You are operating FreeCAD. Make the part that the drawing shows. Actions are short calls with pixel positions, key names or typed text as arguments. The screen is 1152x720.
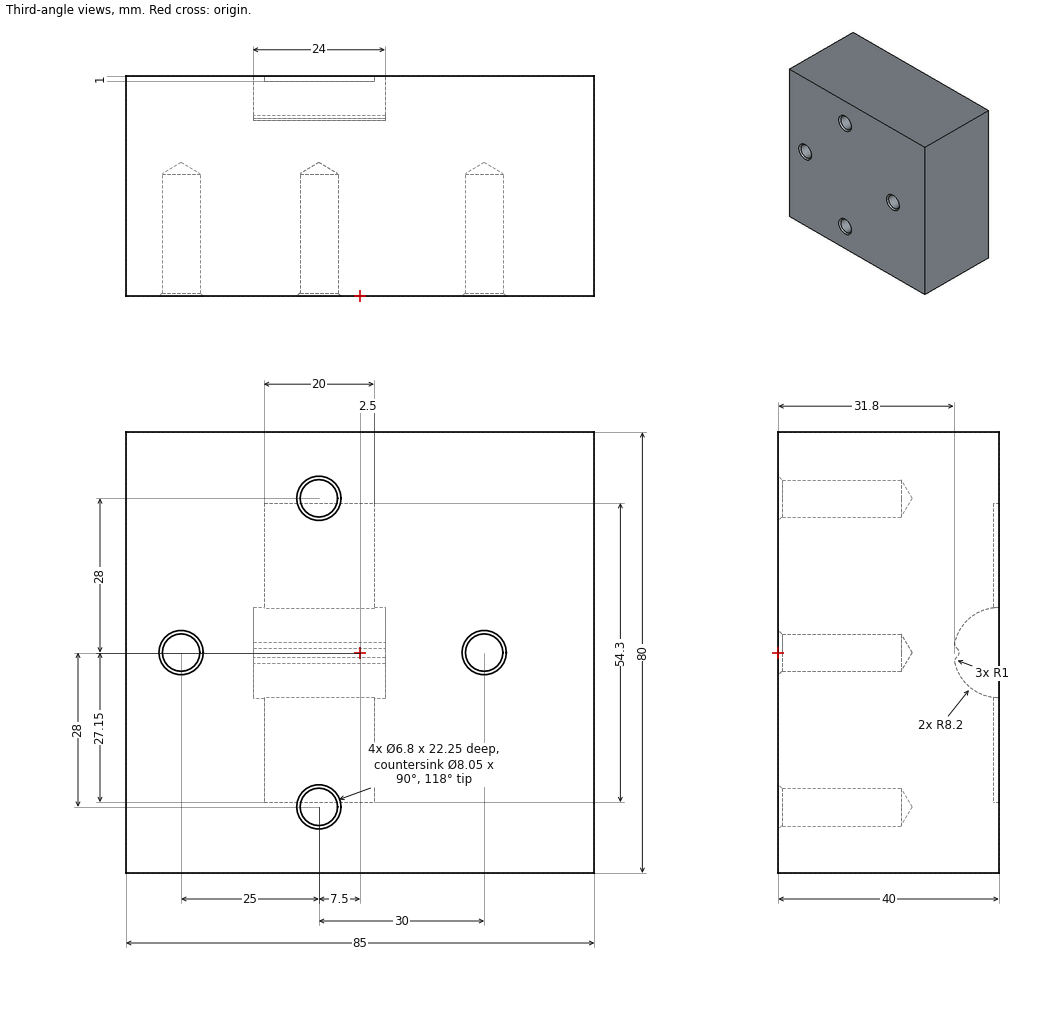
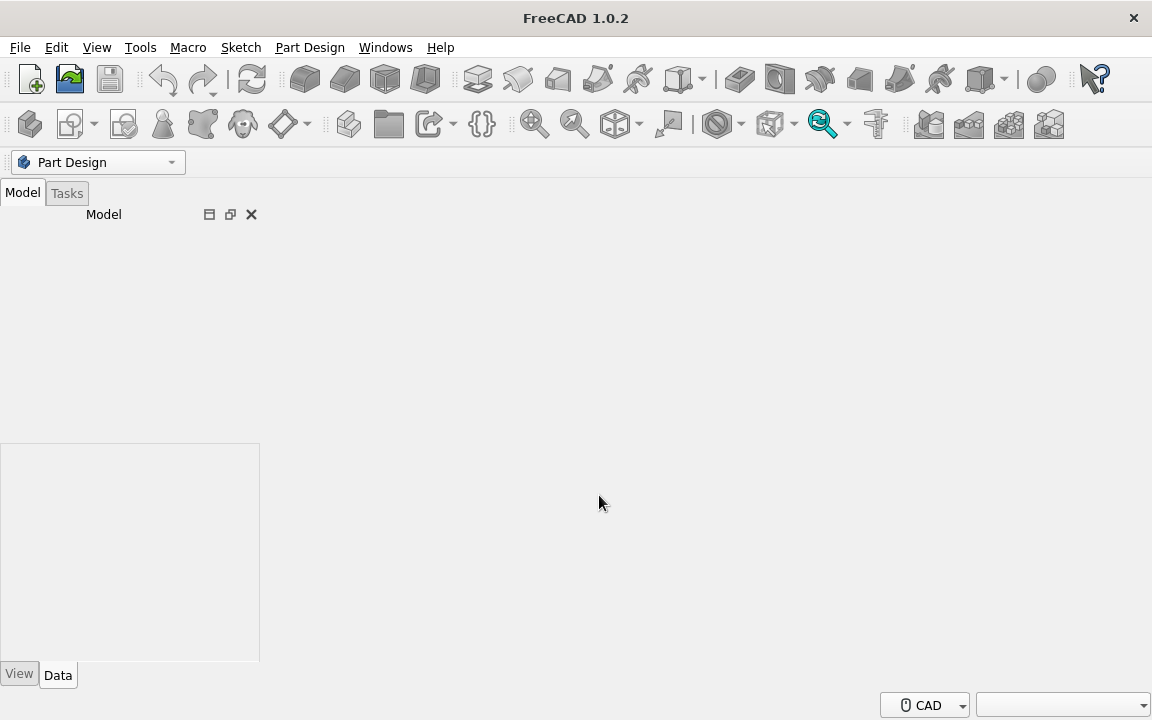
click(30, 80)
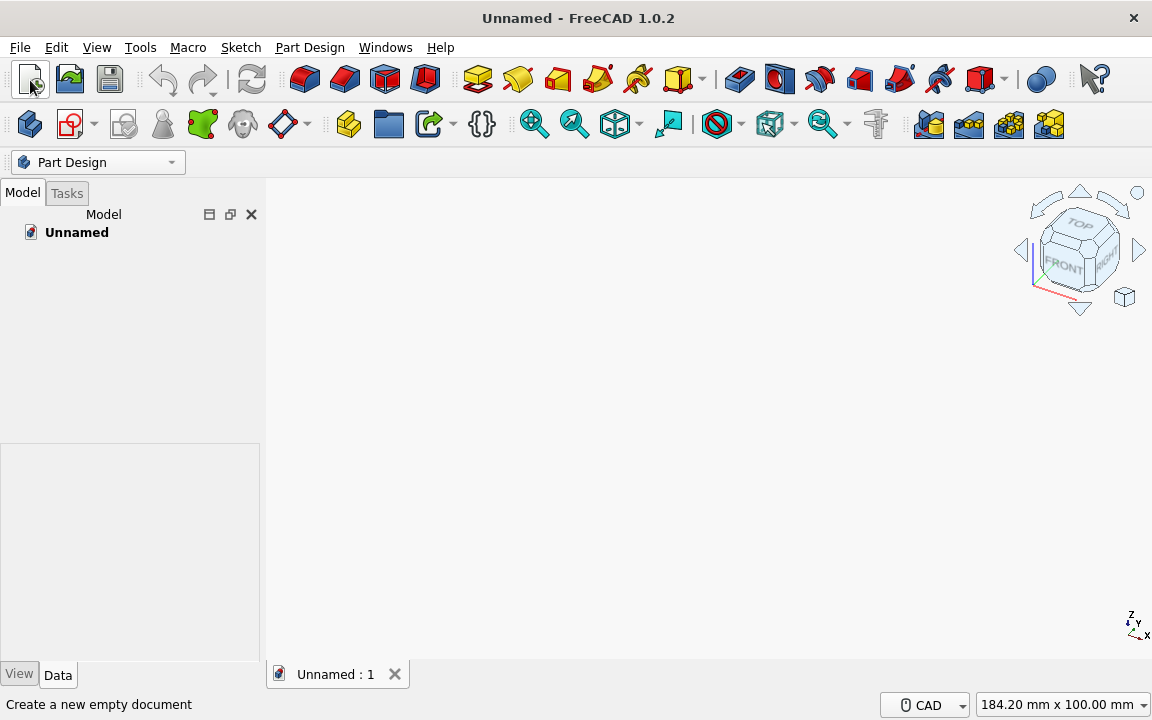
click(70, 124)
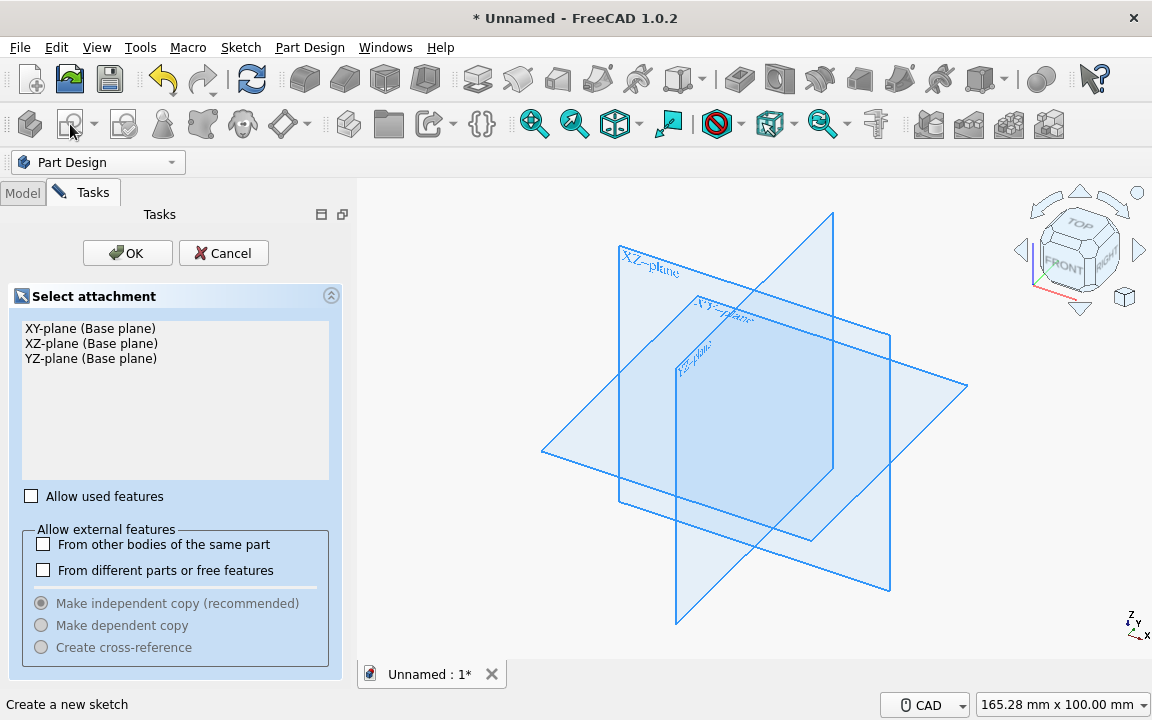
click(82, 344)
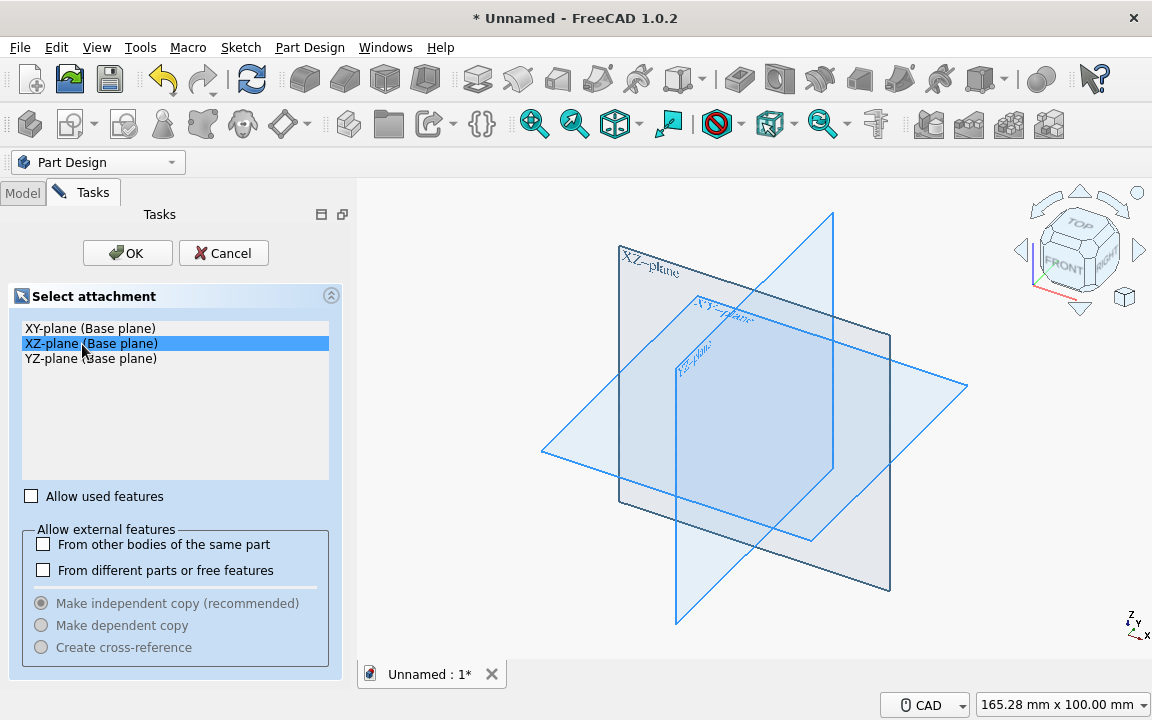
click(128, 253)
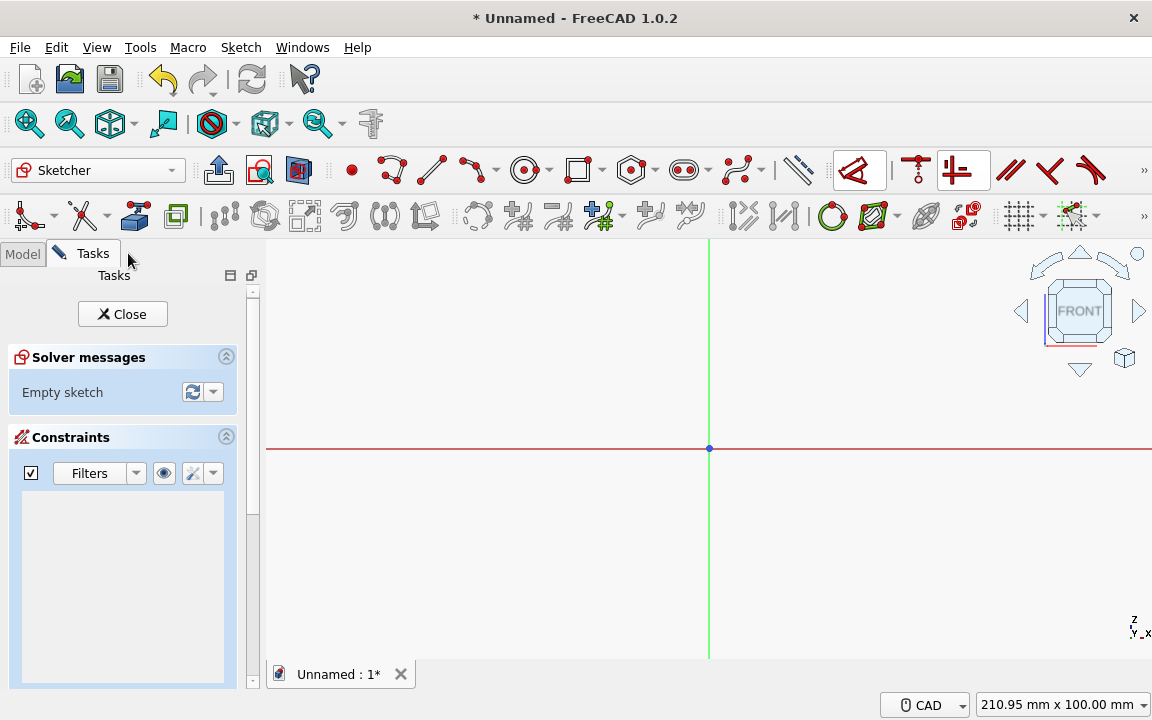
scroll(331, 449, down, 1)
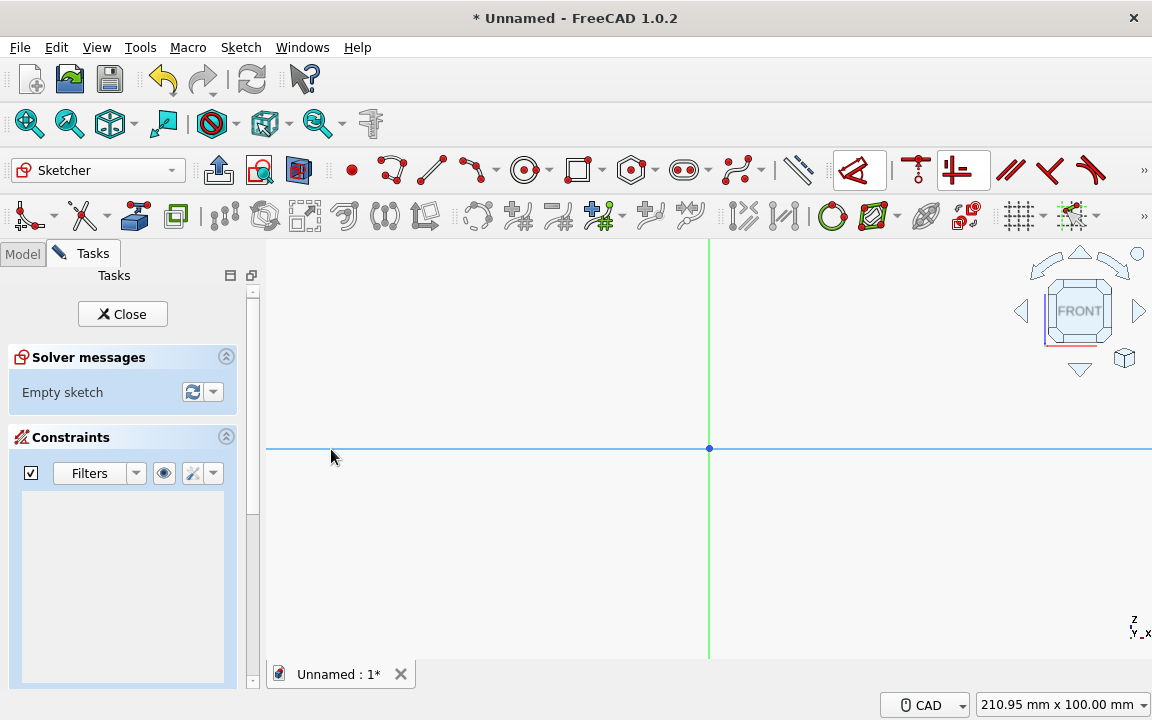
click(604, 170)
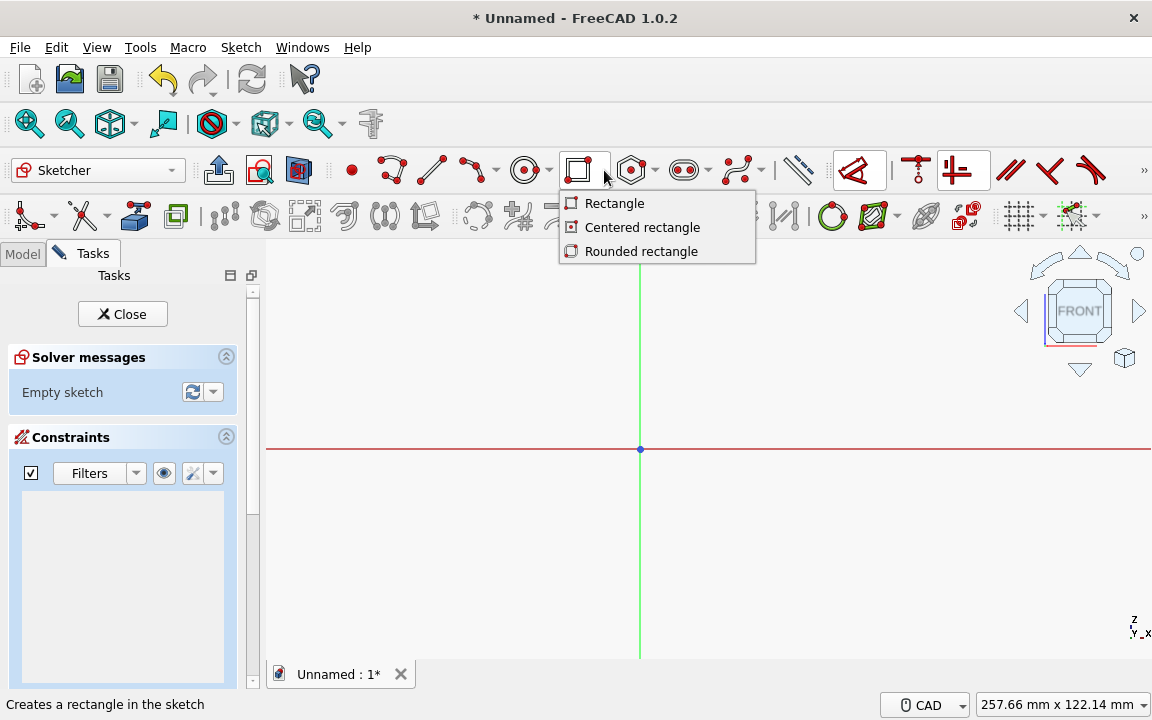
click(658, 227)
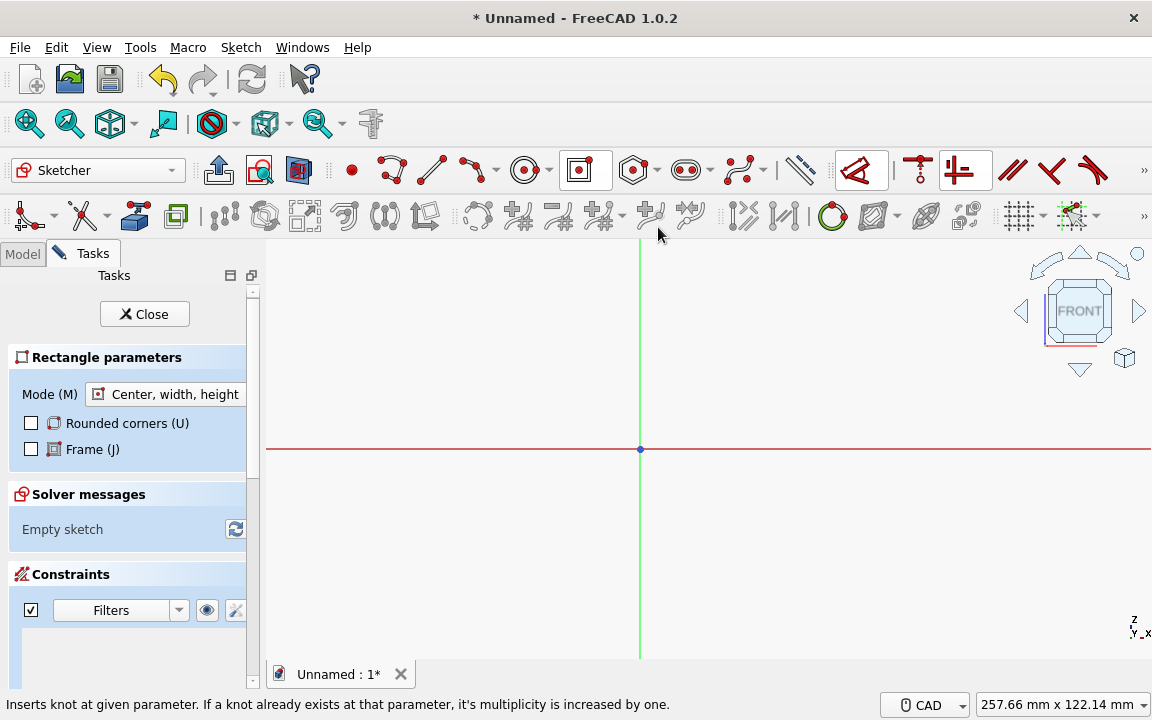
click(640, 449)
move(787, 312)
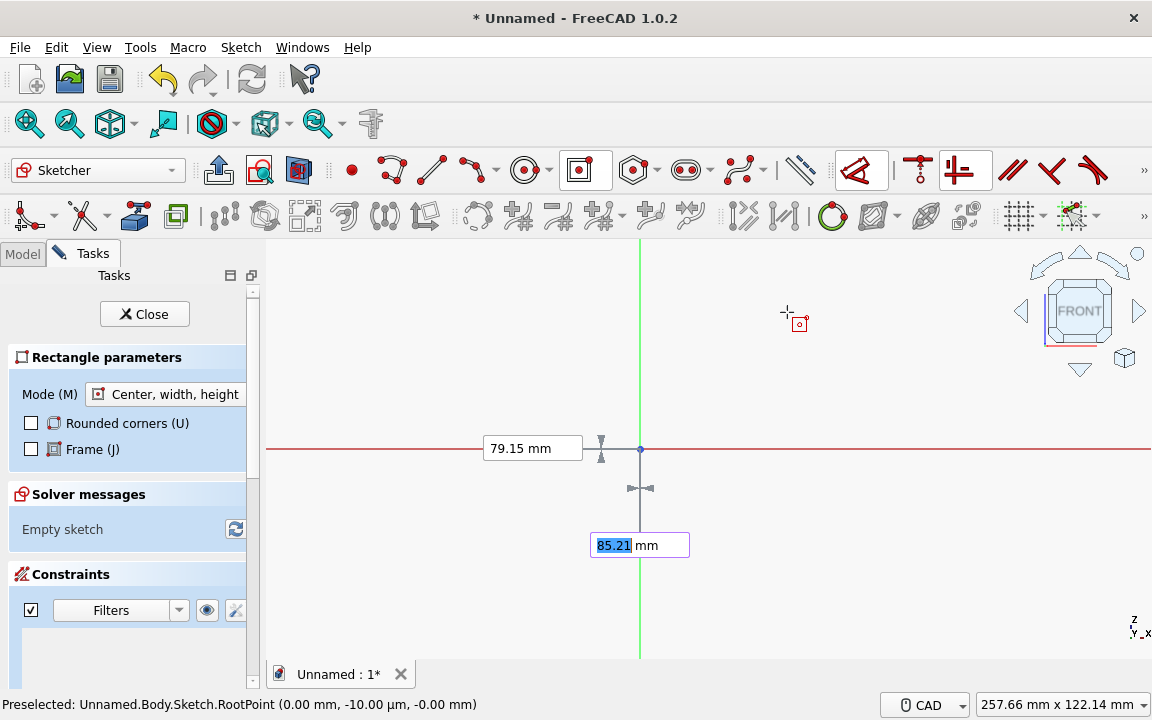
text(85)
key(Tab)
text(80)
key(Return)
key(Escape)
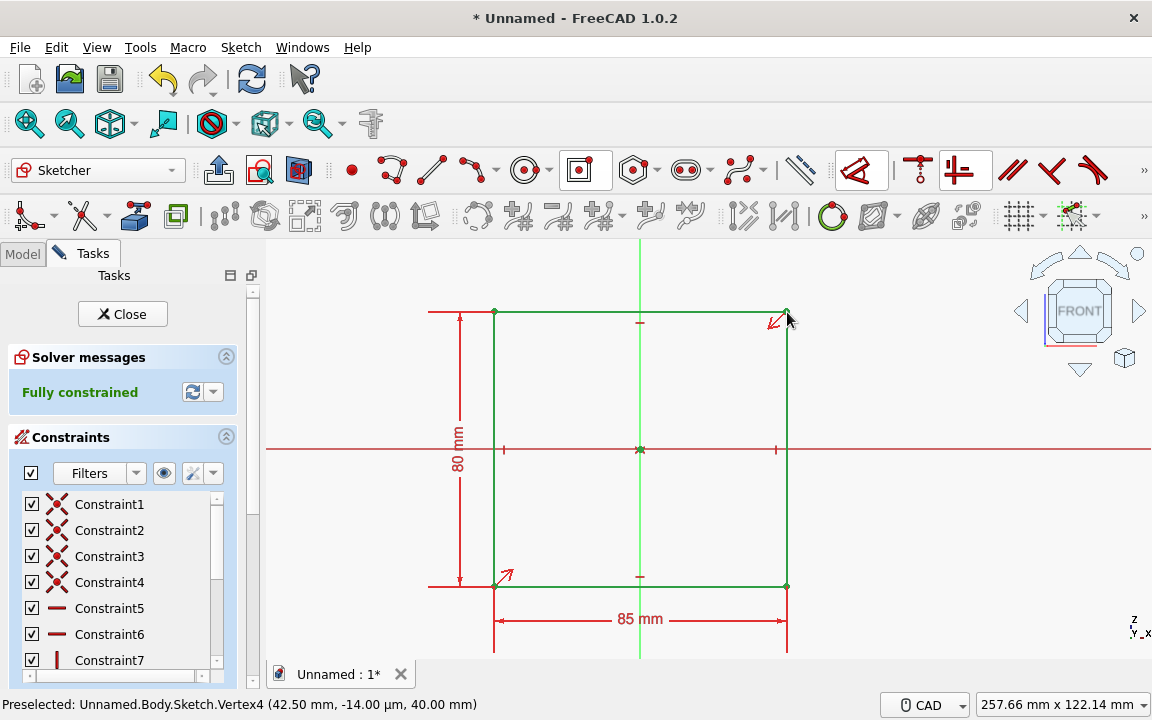
click(123, 314)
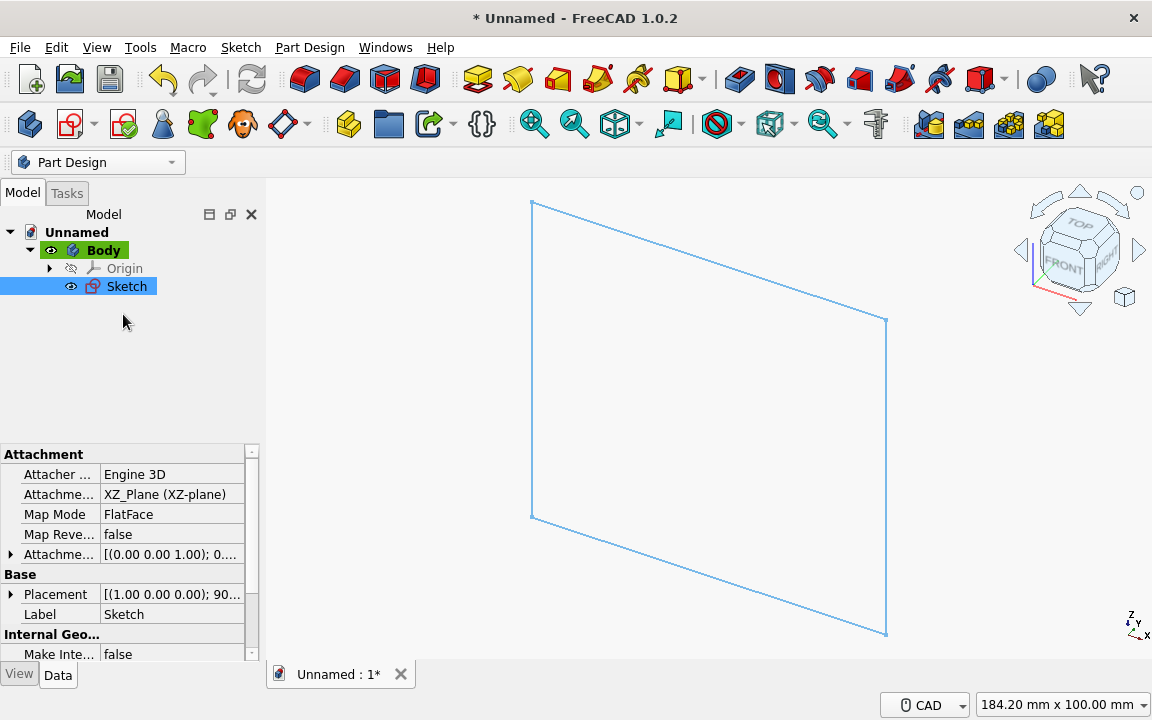
click(478, 80)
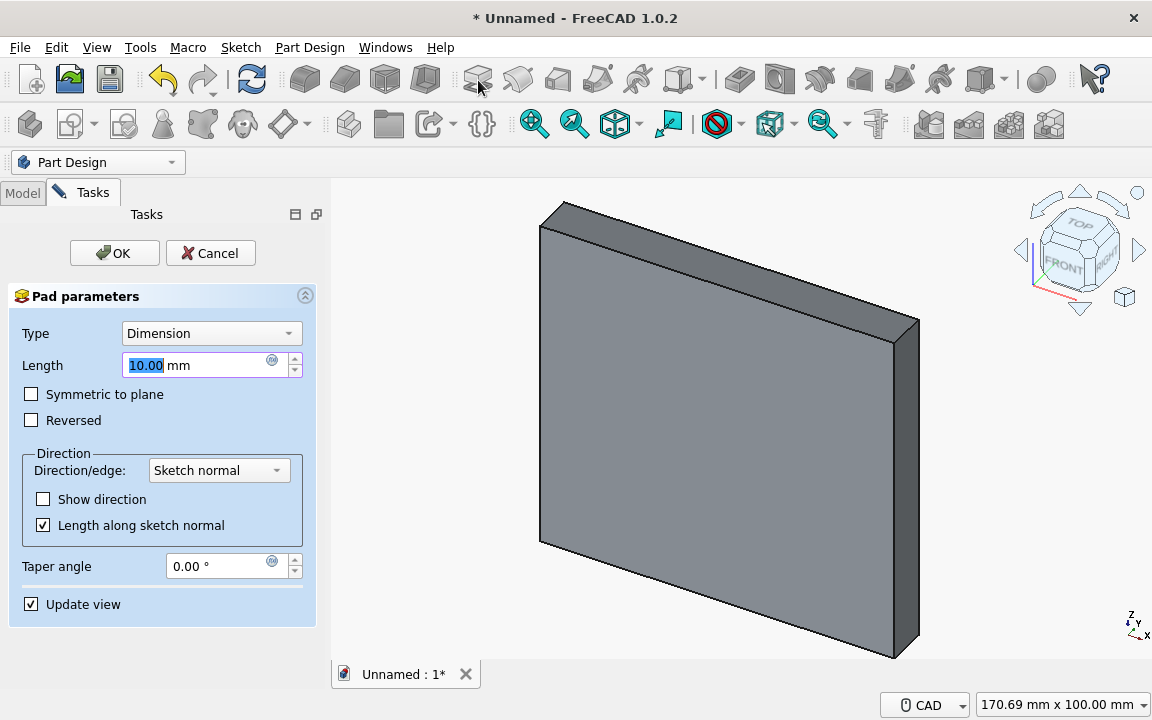
text(40)
key(Tab)